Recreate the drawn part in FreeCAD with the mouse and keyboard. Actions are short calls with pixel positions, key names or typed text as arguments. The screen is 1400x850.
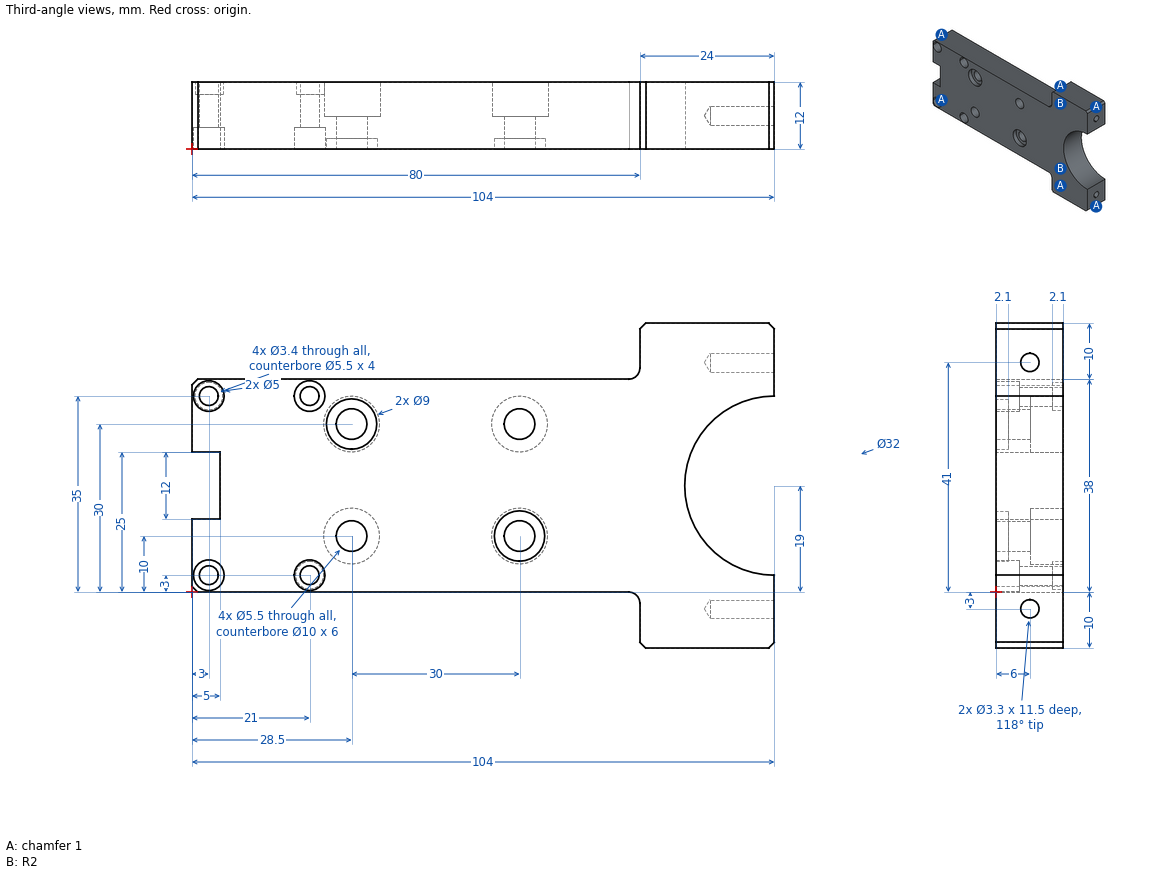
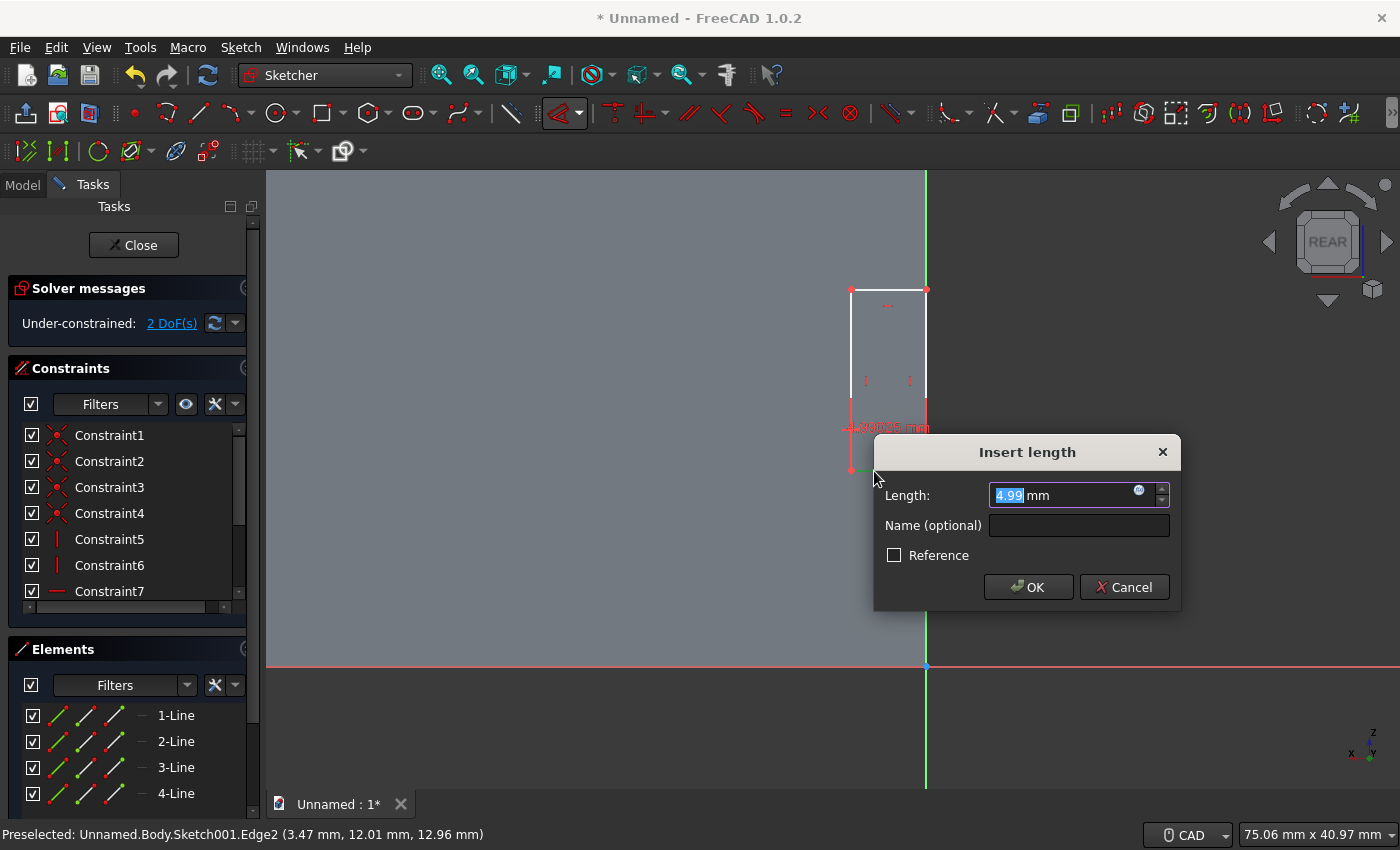
text(5)
key(Return)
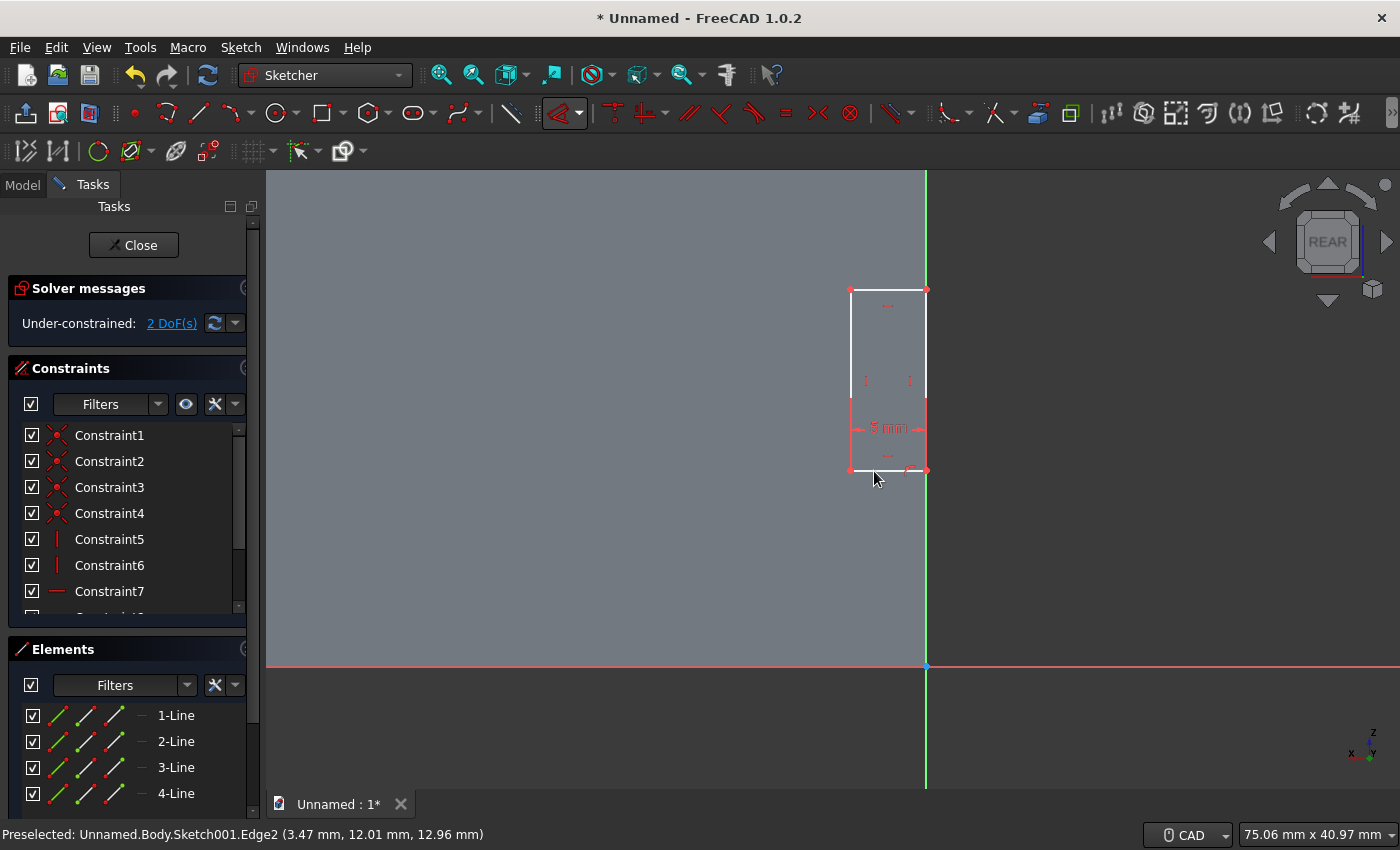
click(851, 344)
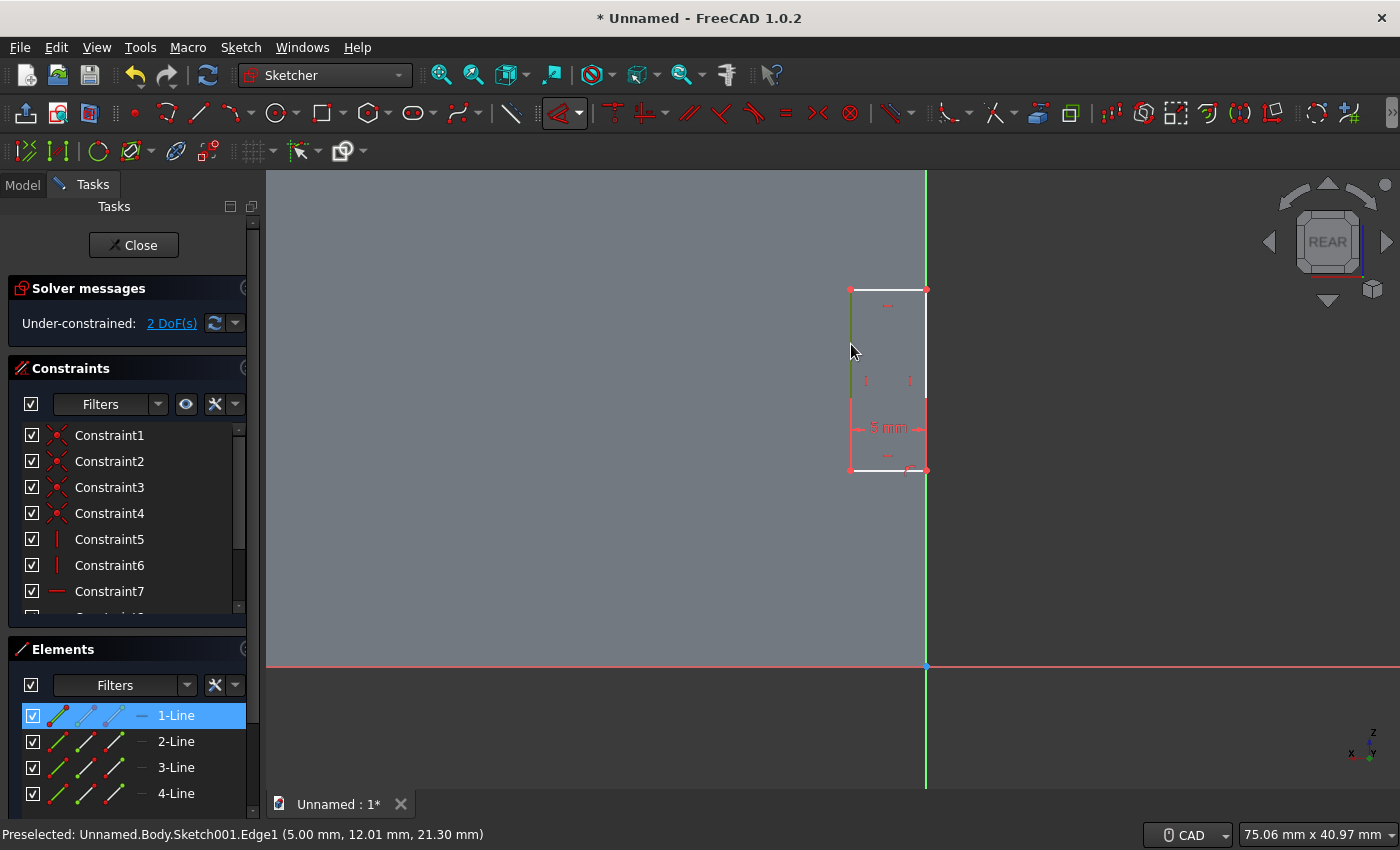
click(582, 114)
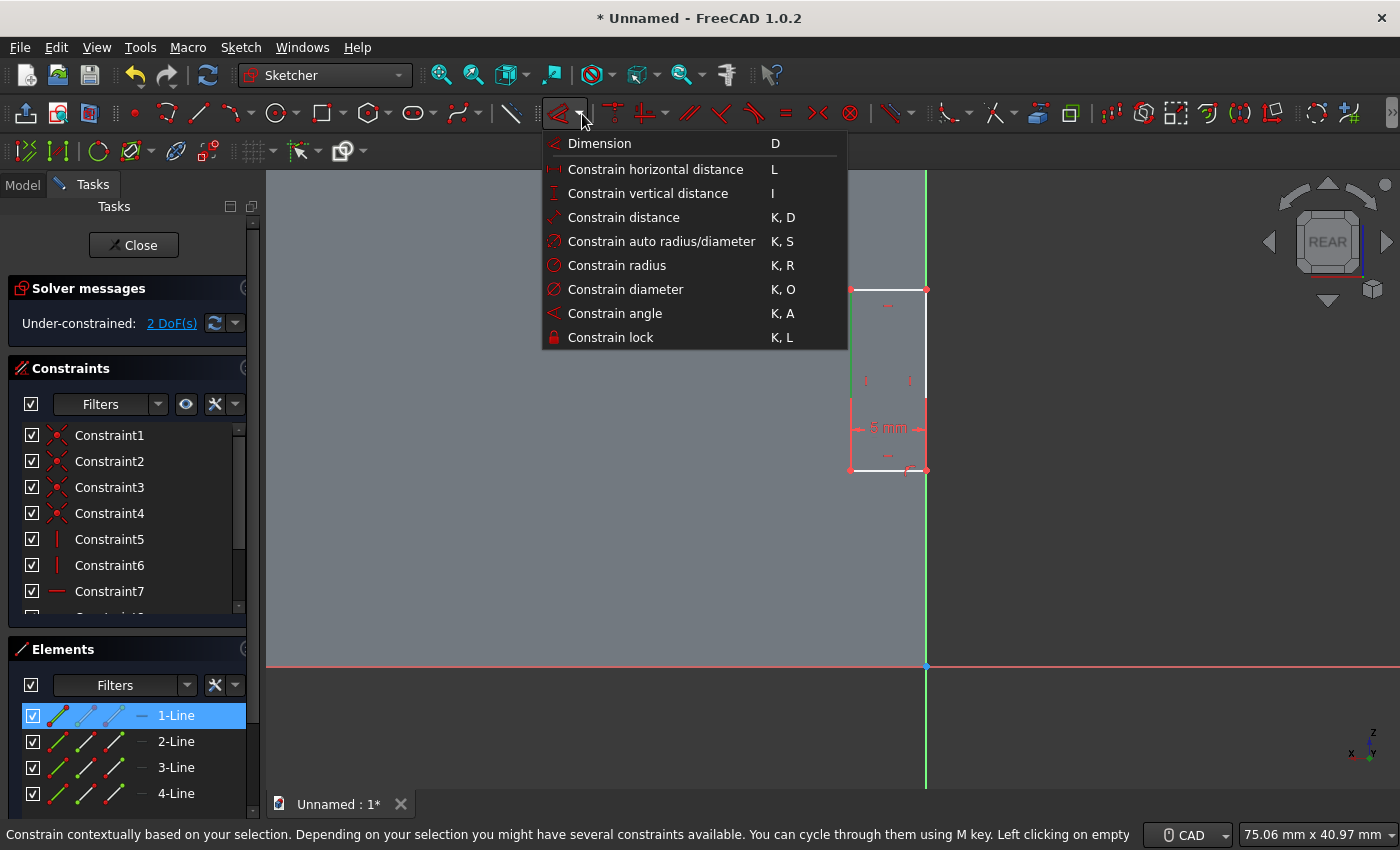
click(695, 193)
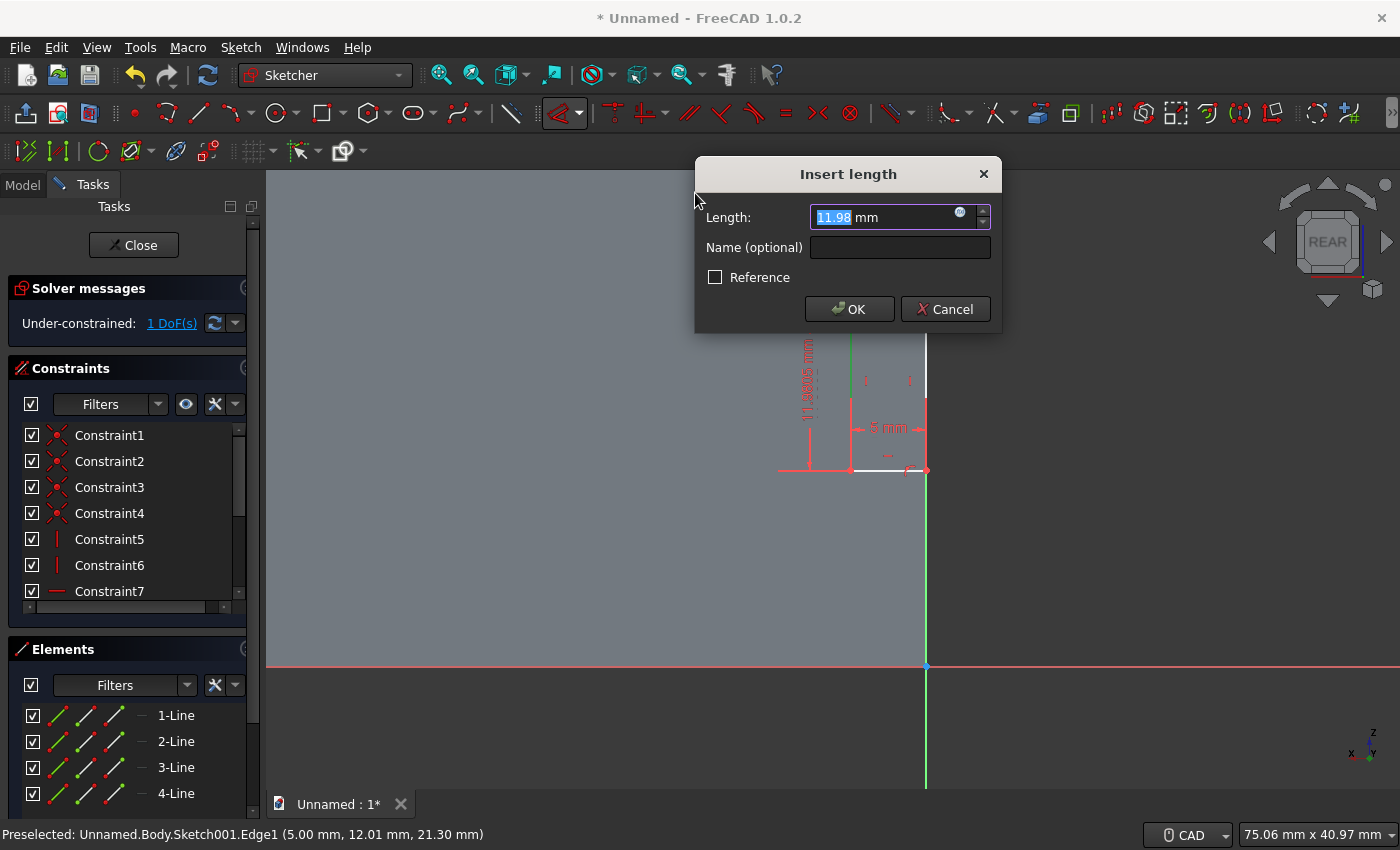
text(12)
key(Return)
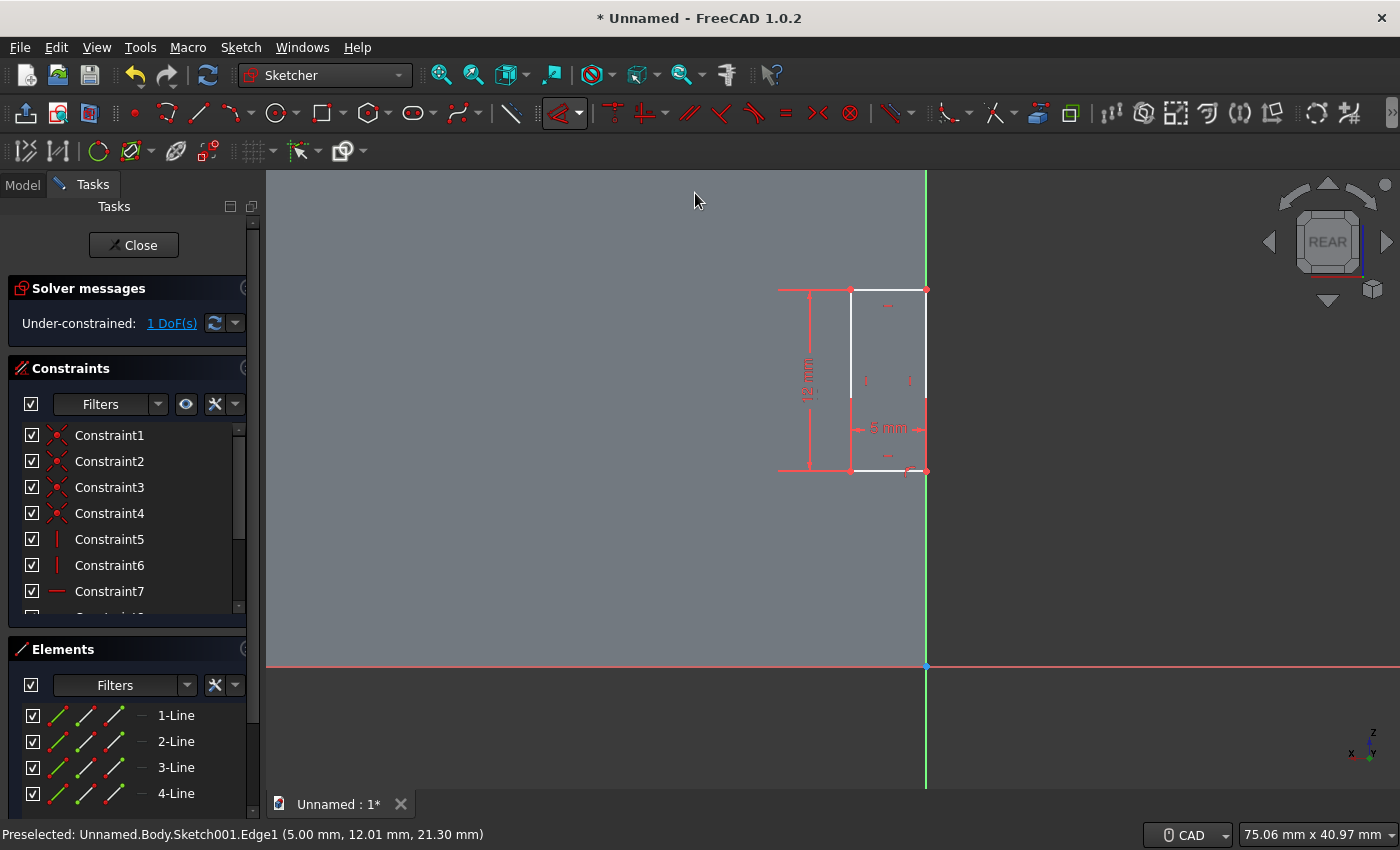
click(851, 290)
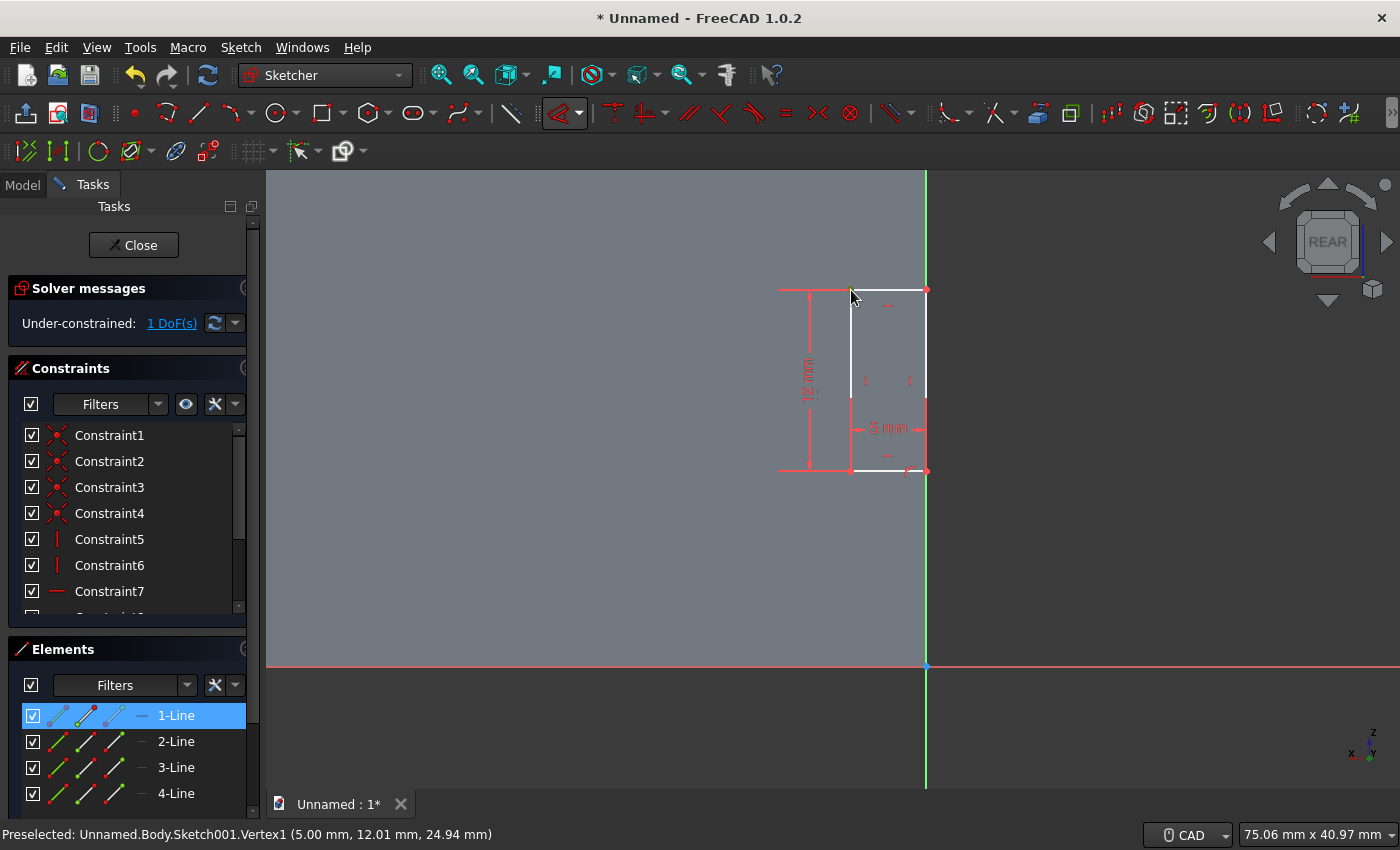
click(582, 114)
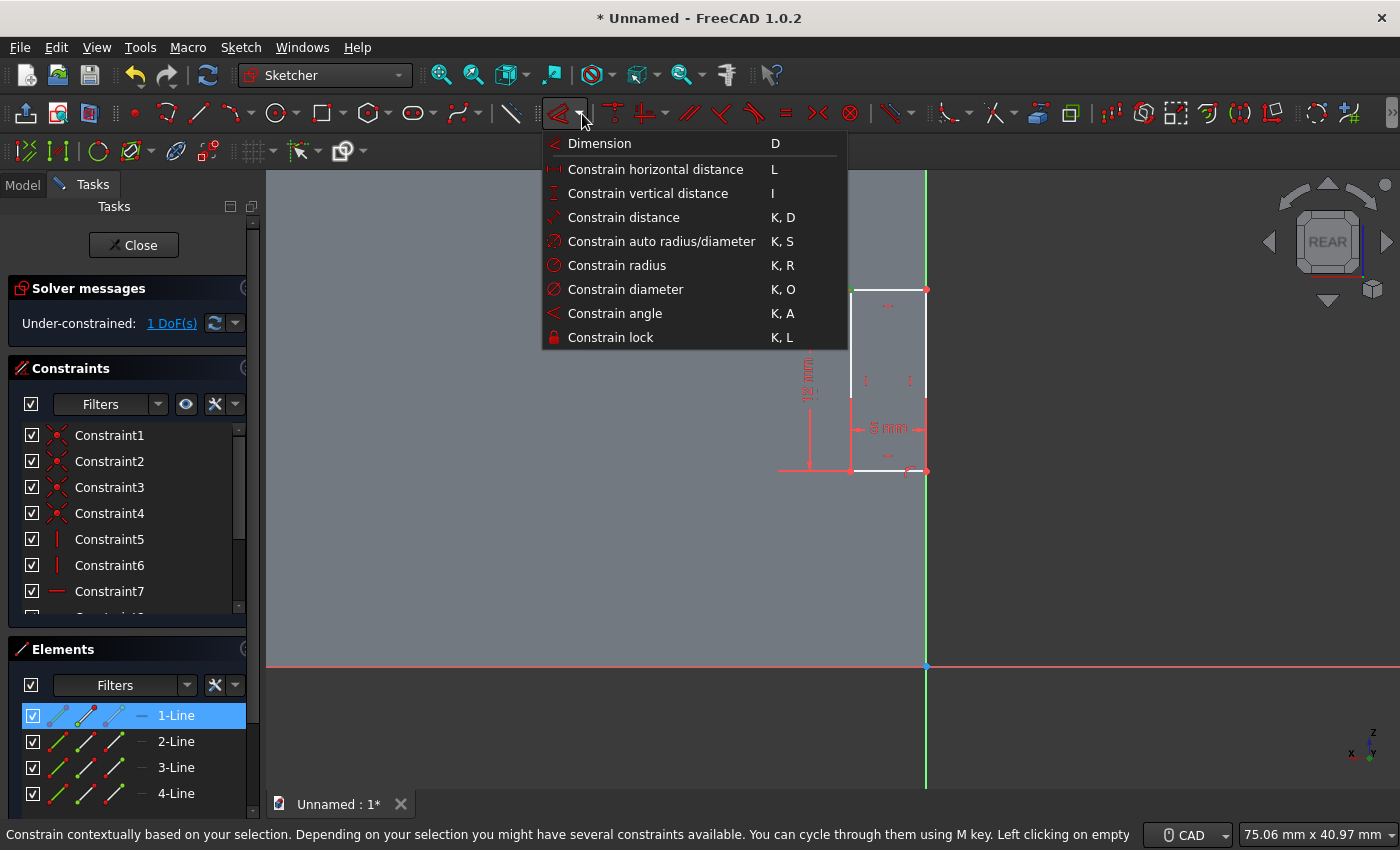
click(695, 193)